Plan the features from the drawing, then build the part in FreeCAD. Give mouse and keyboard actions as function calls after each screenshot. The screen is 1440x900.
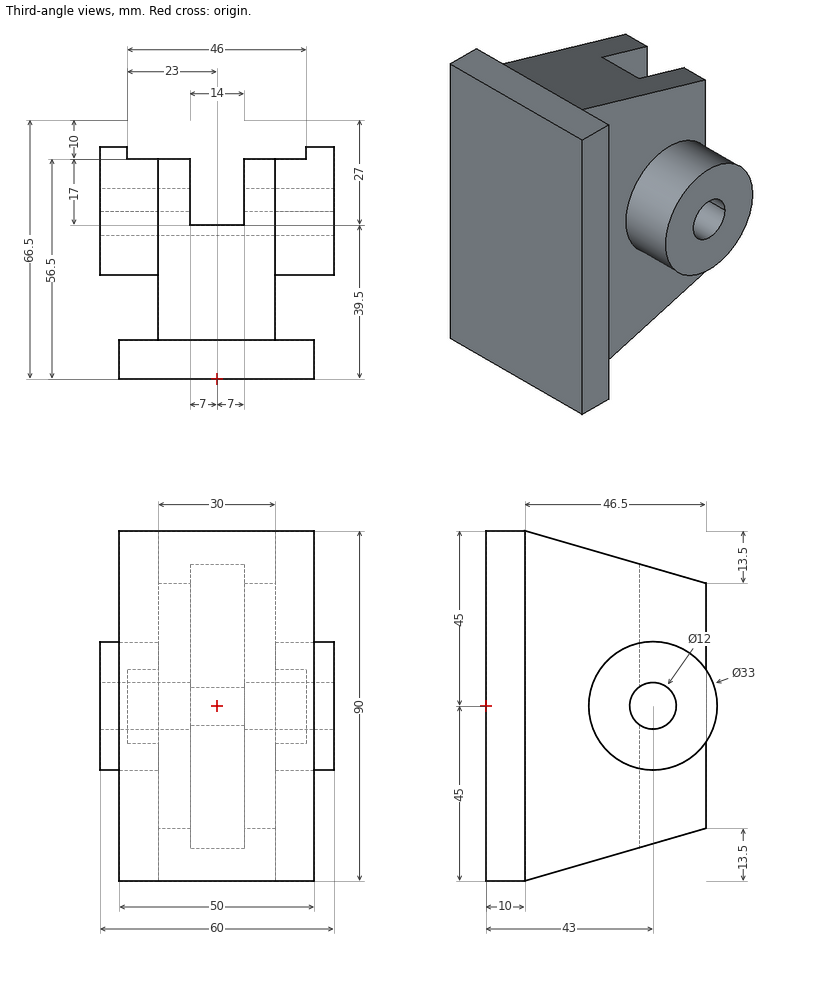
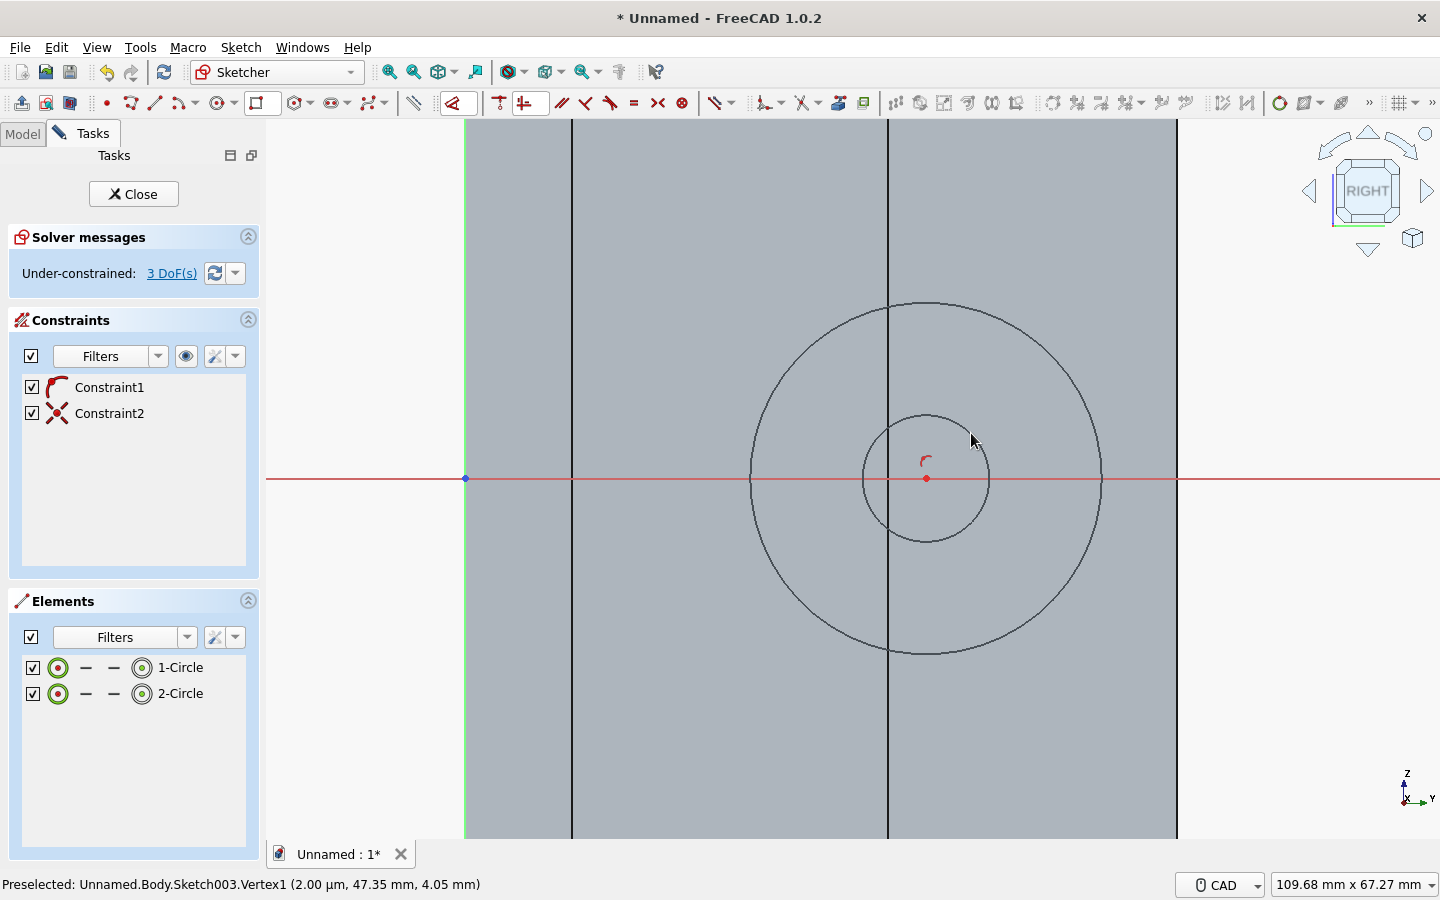
click(1050, 354)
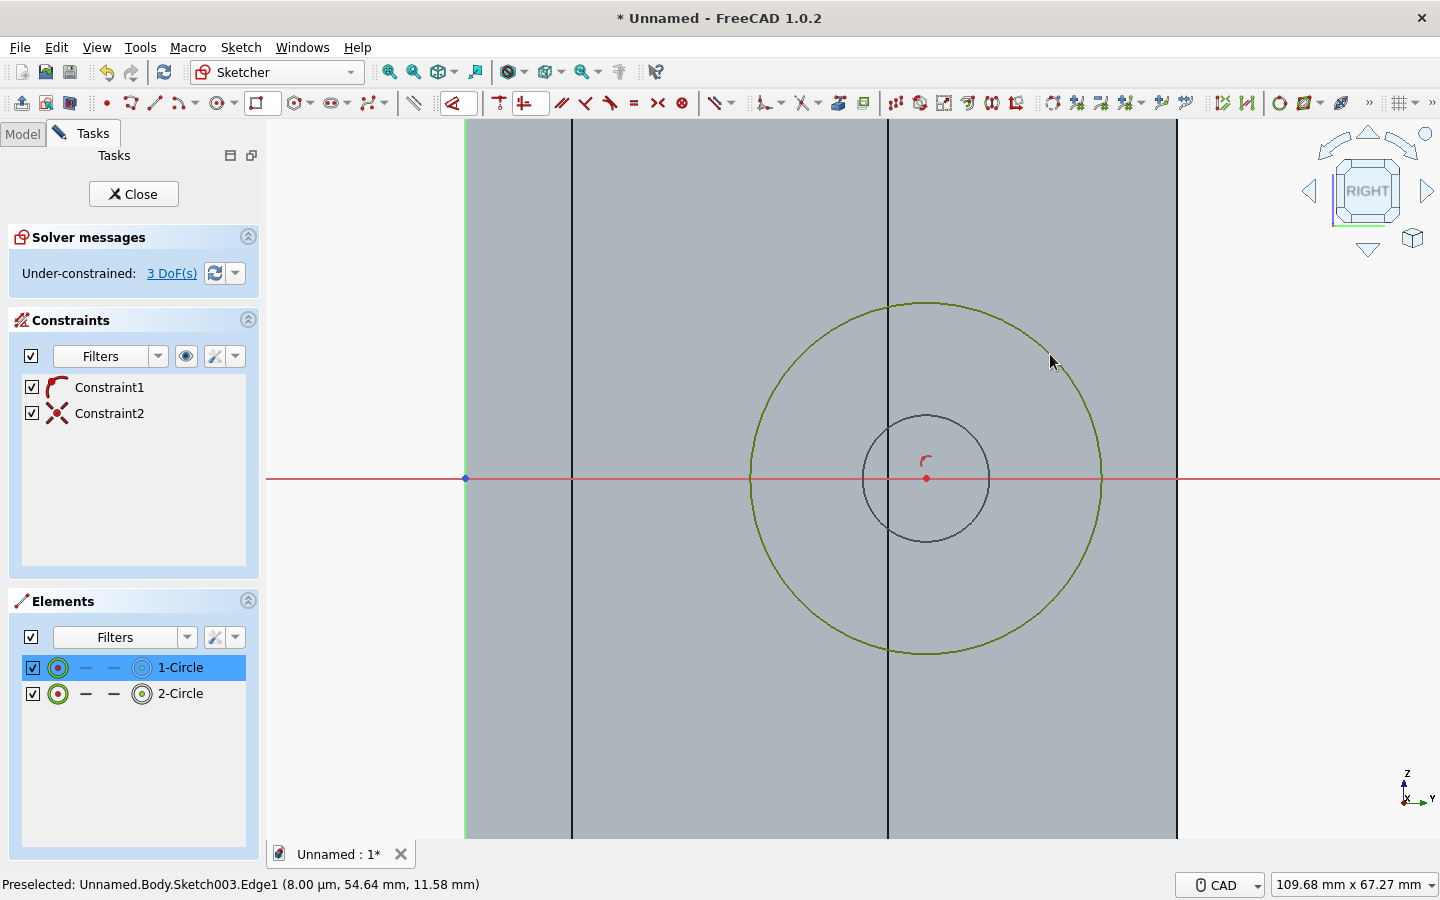
click(472, 104)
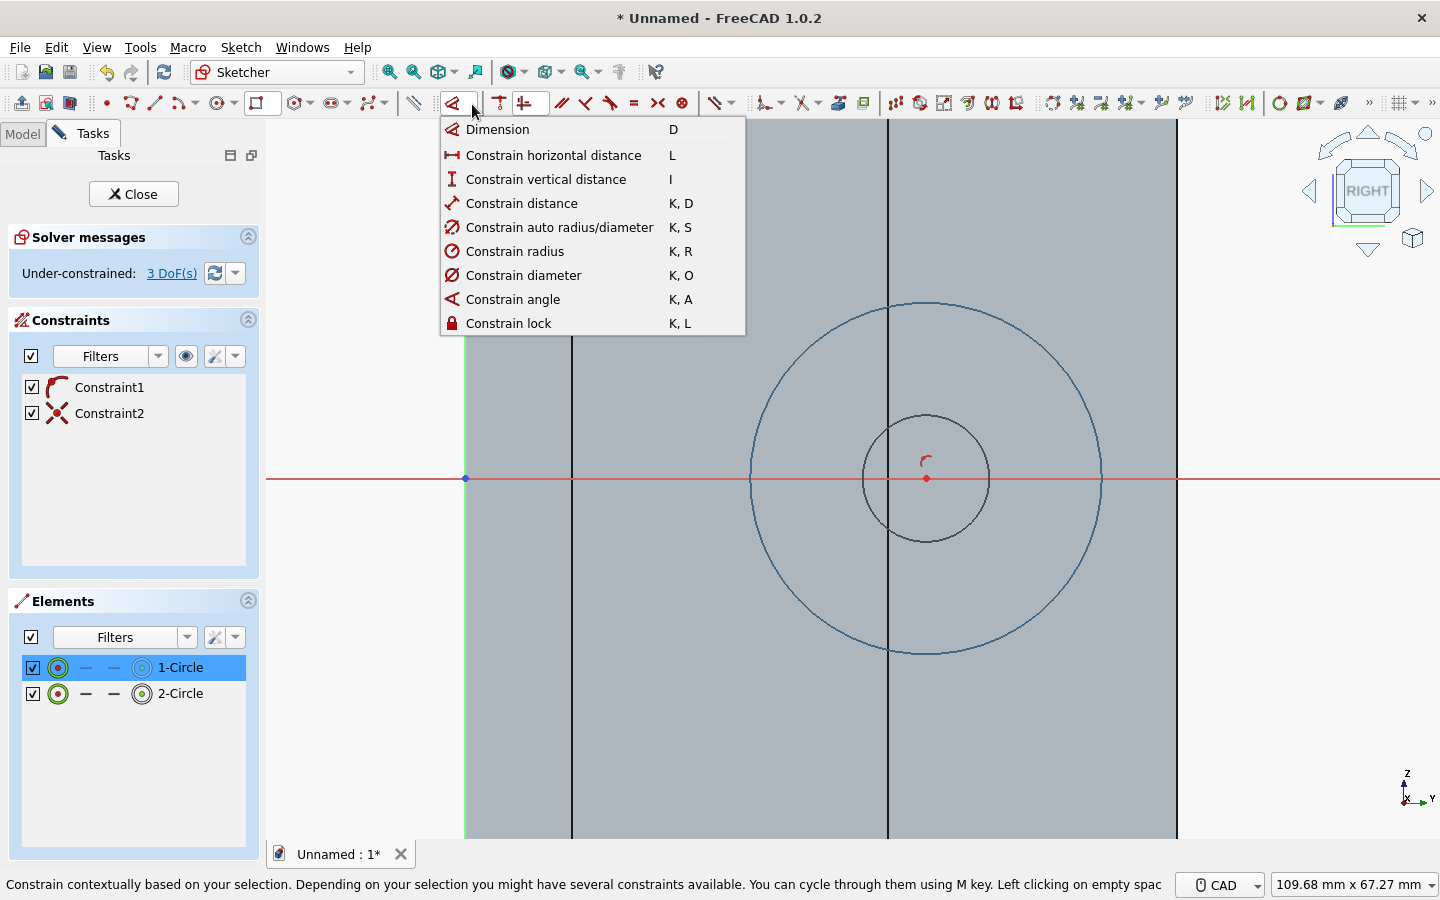
click(593, 275)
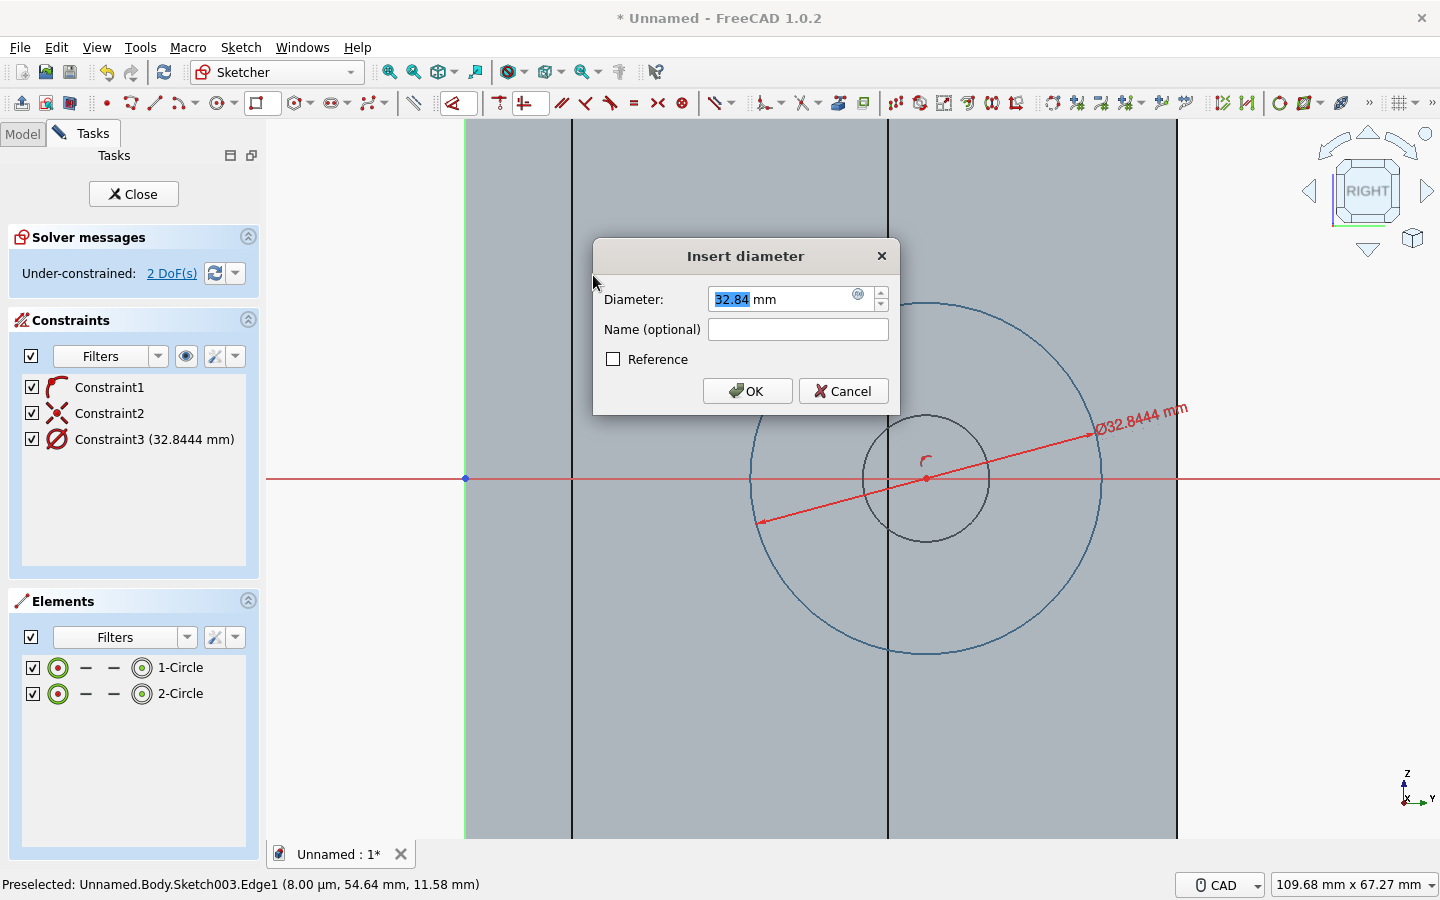
text(33)
key(Return)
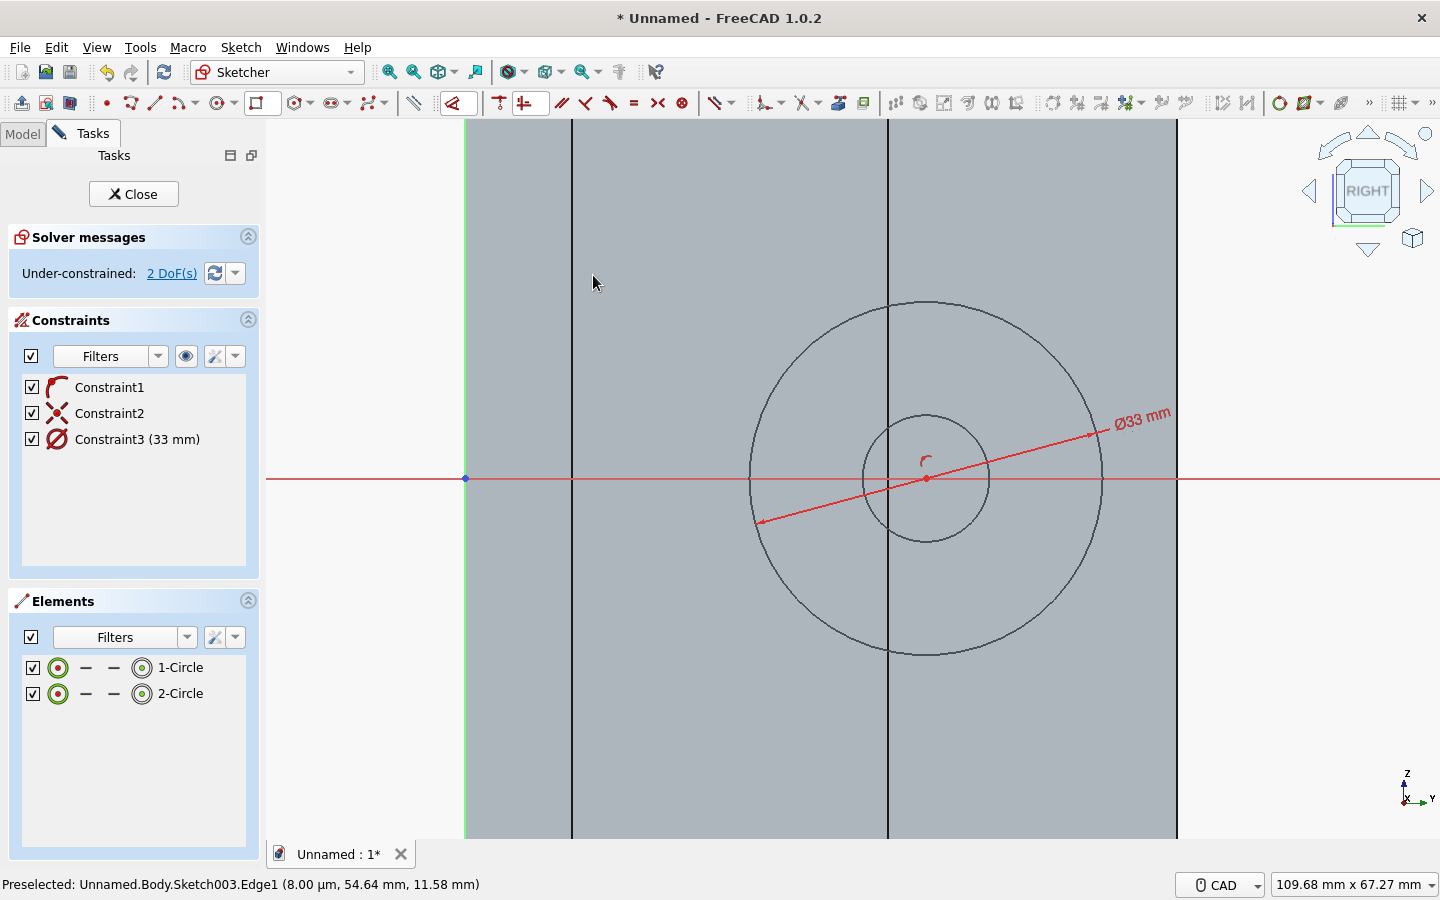
click(971, 434)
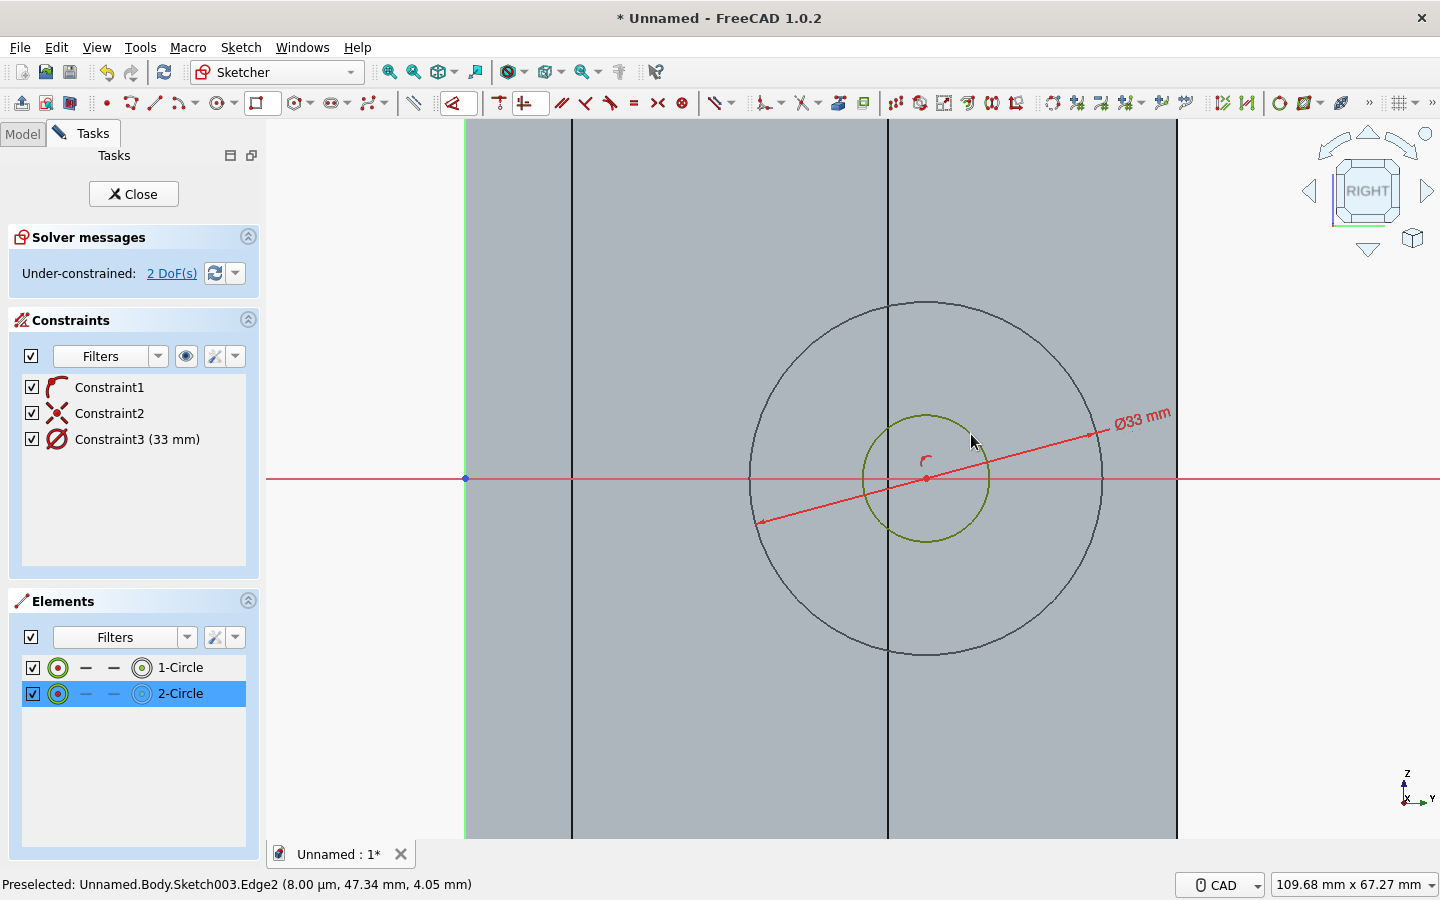
click(472, 104)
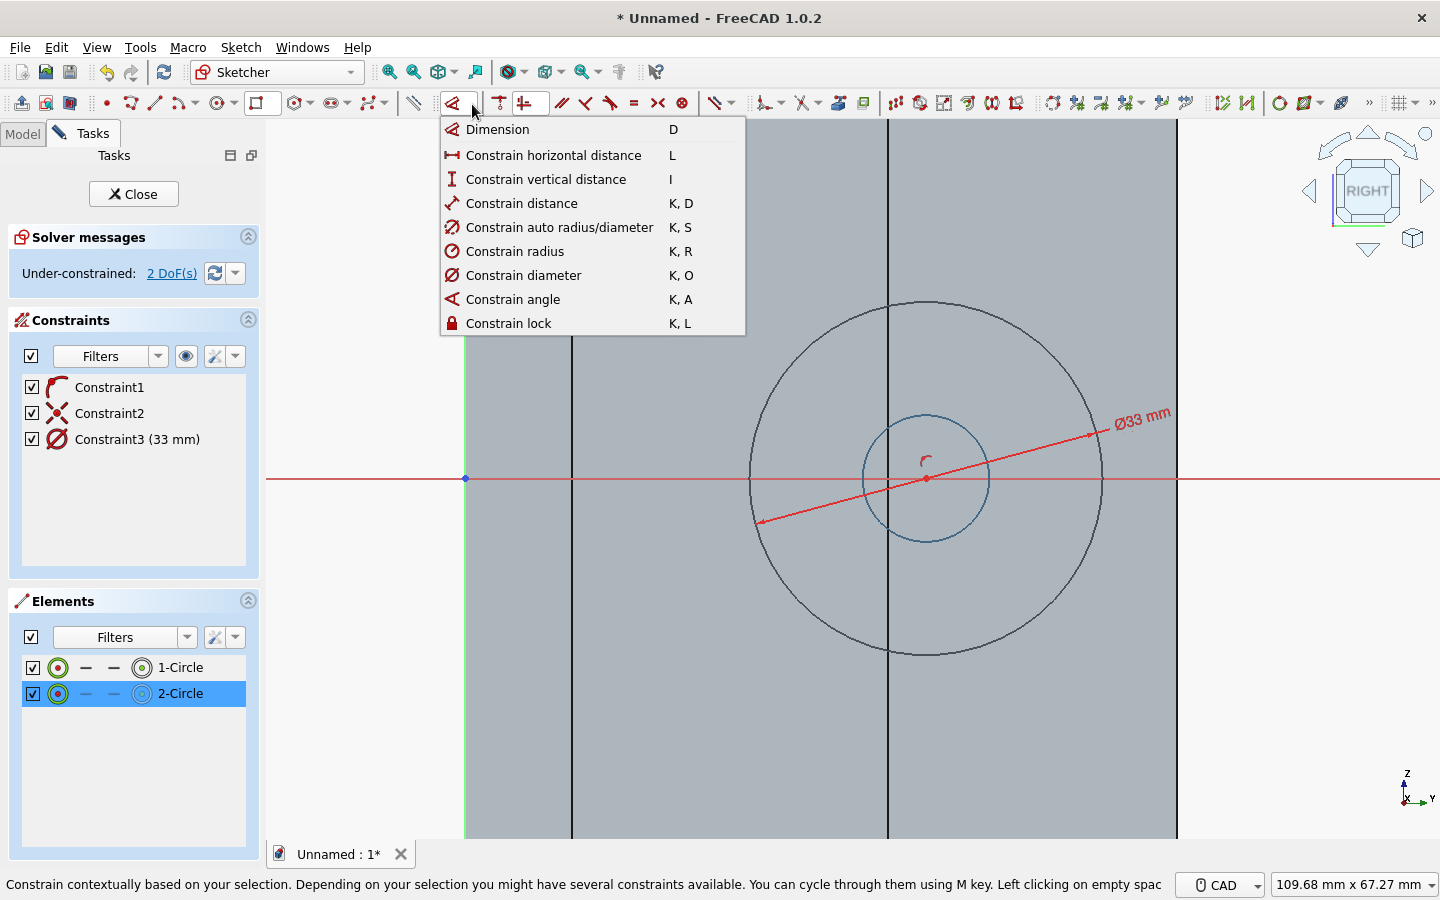
click(593, 275)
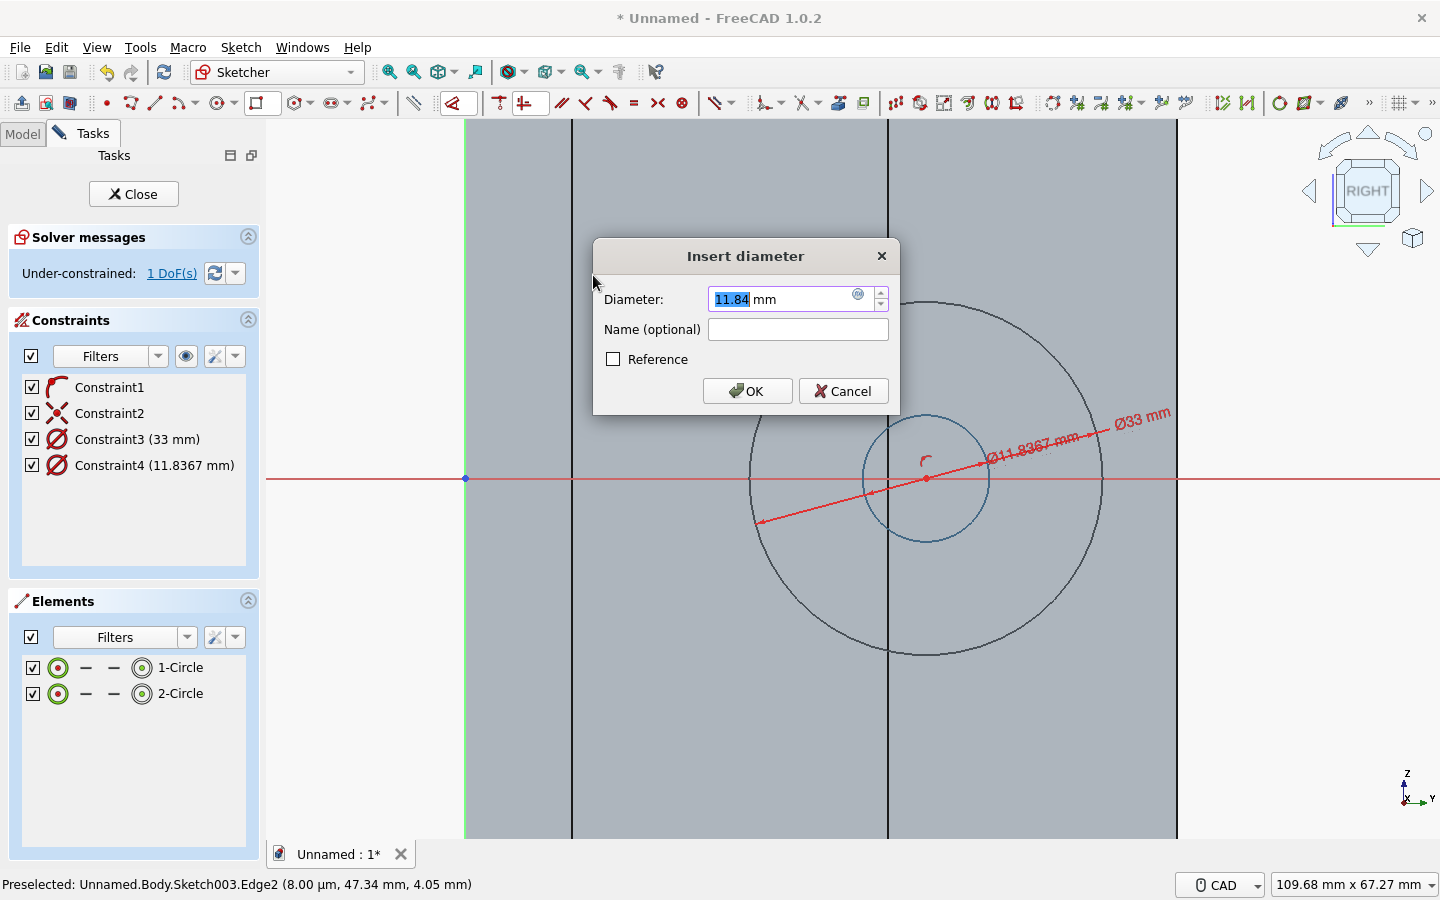
text(12)
key(Return)